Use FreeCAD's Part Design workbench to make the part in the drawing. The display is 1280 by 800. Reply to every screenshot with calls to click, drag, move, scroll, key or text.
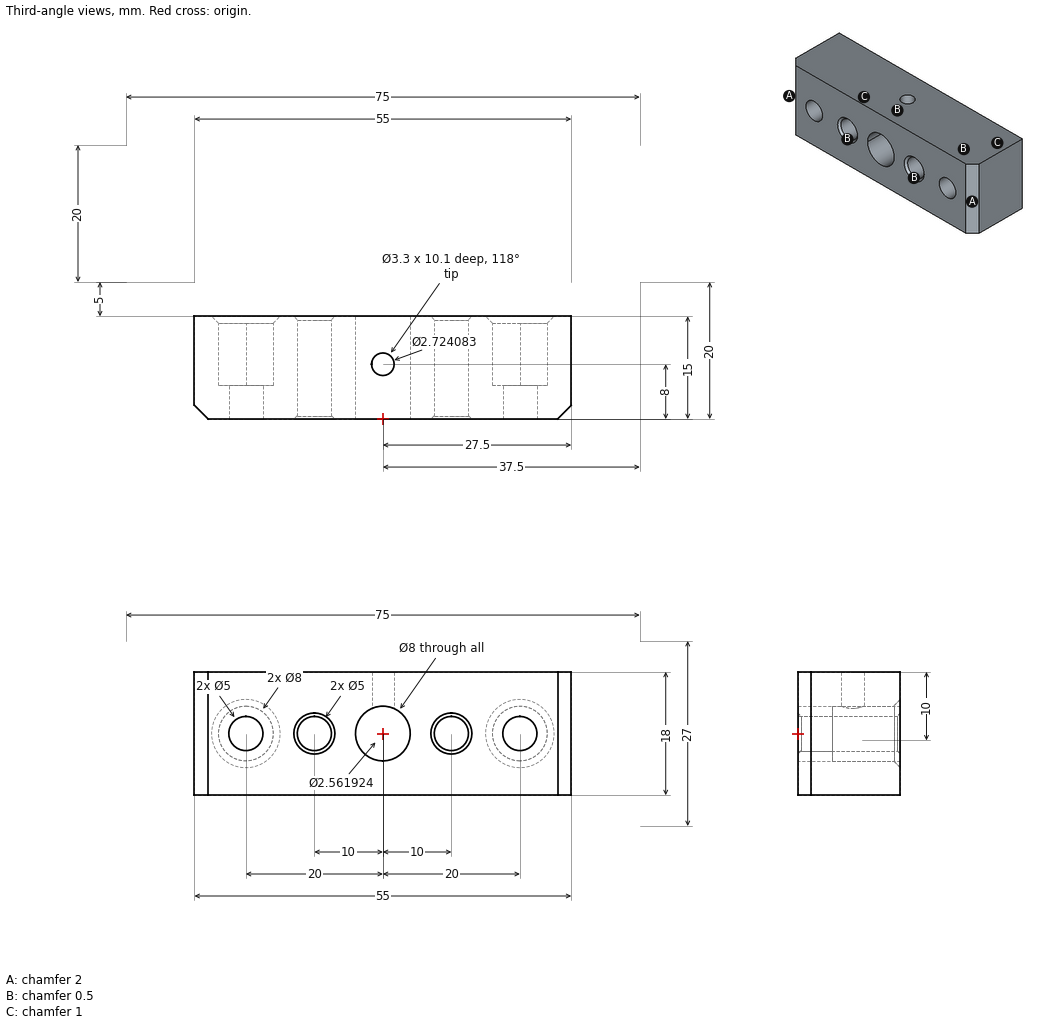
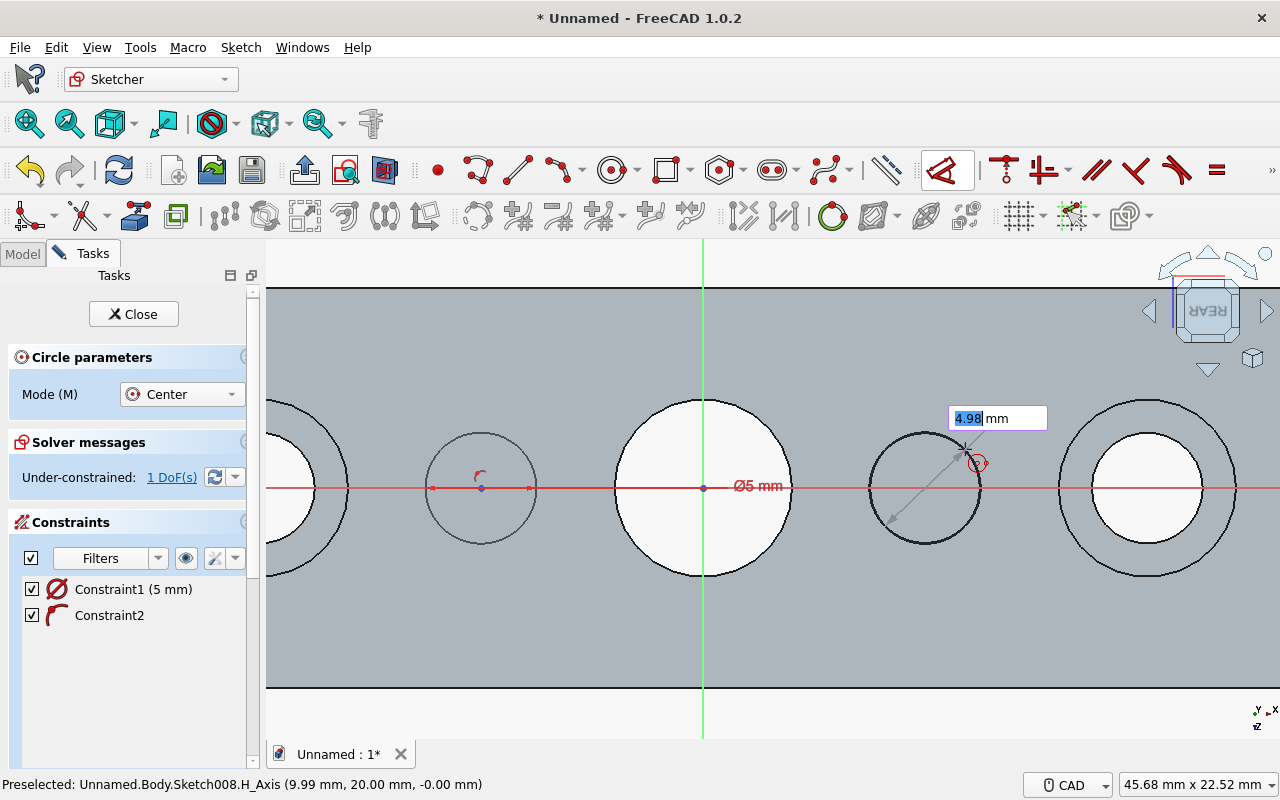
text(5)
key(Return)
key(Escape)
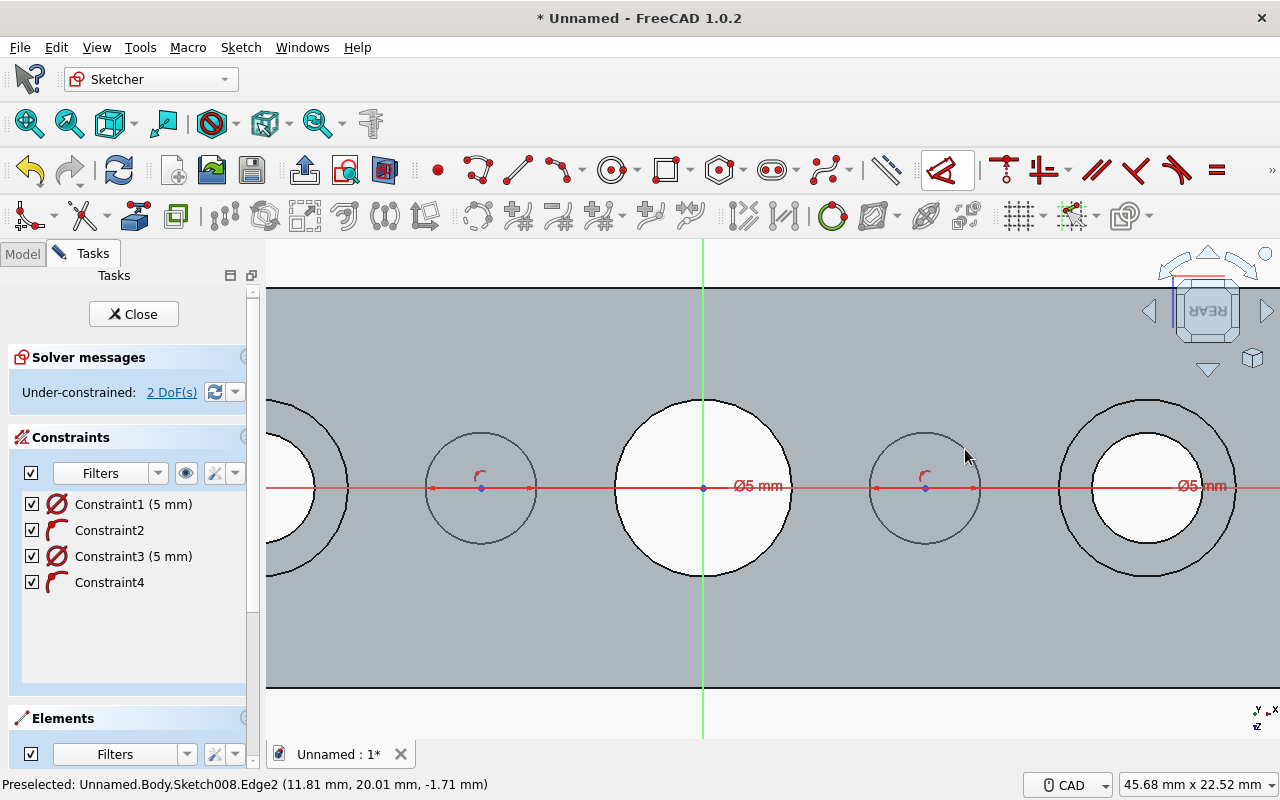
click(481, 488)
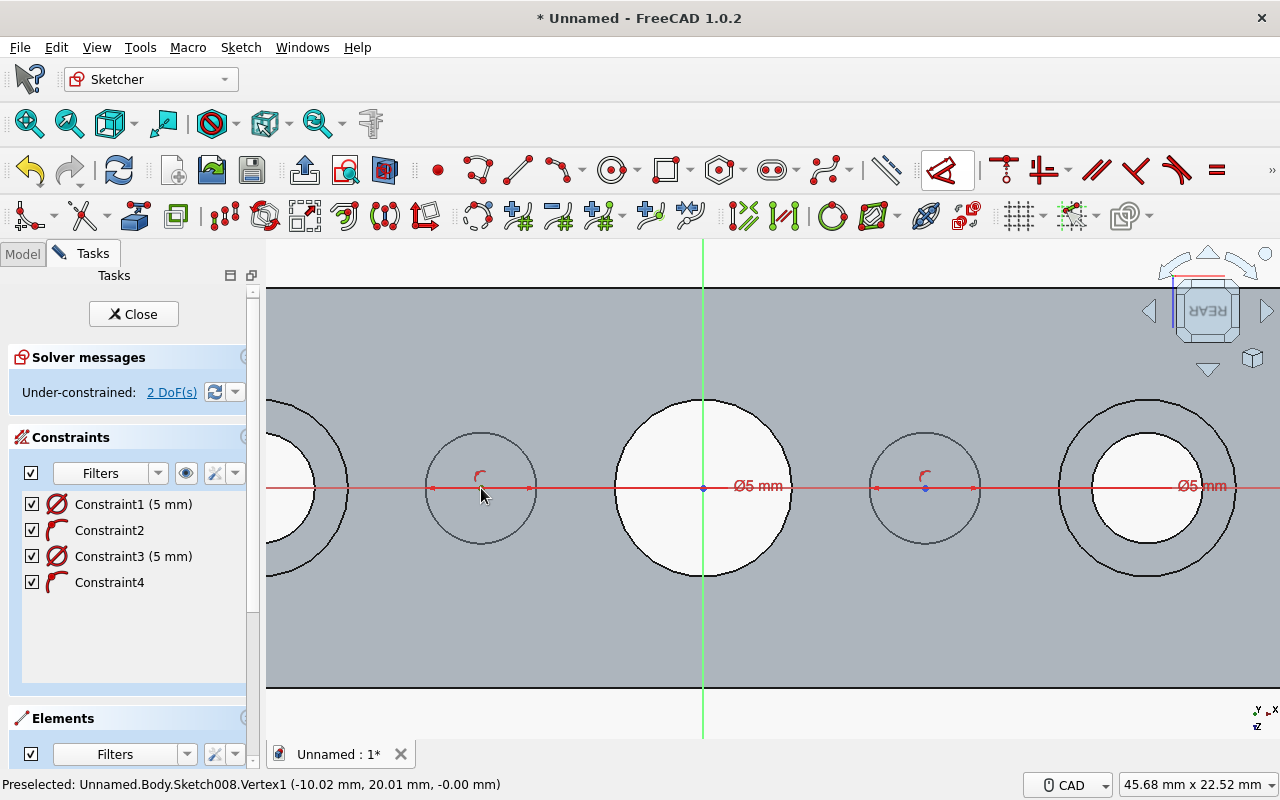
click(968, 170)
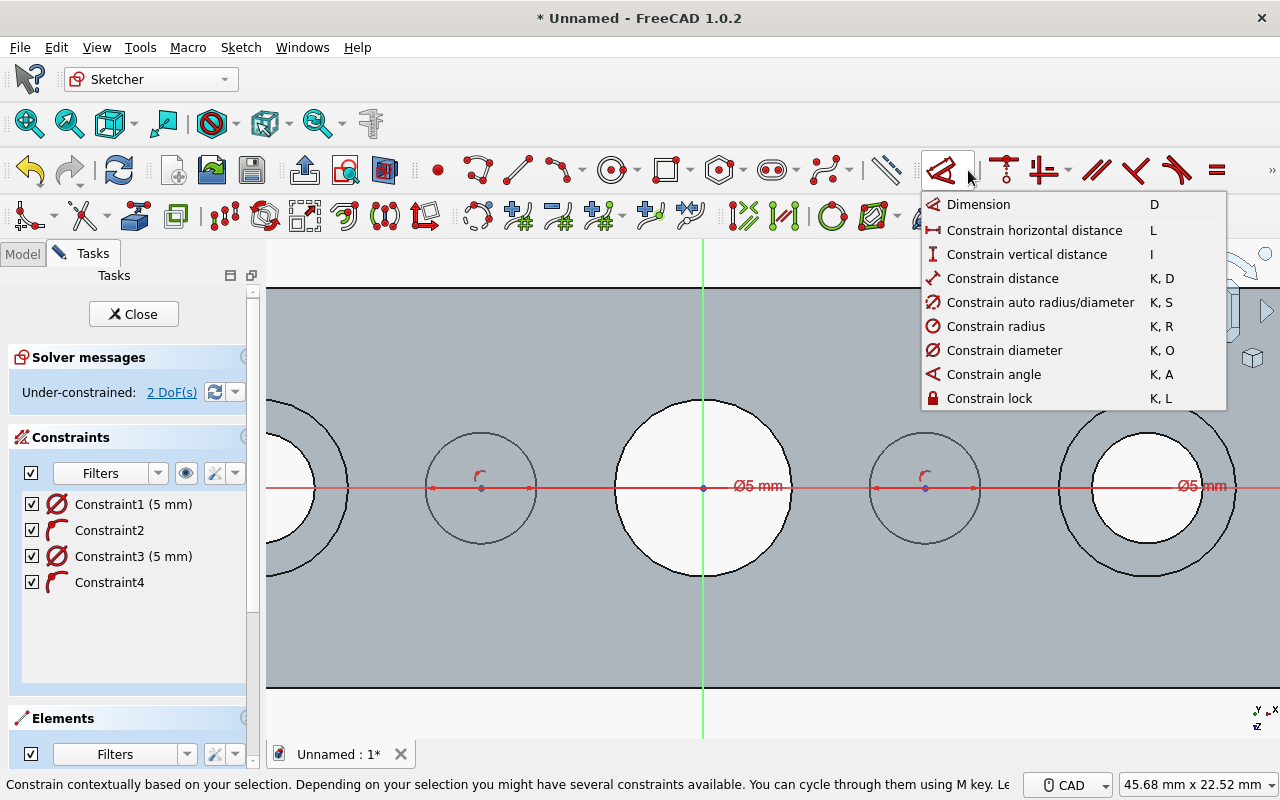
click(1074, 230)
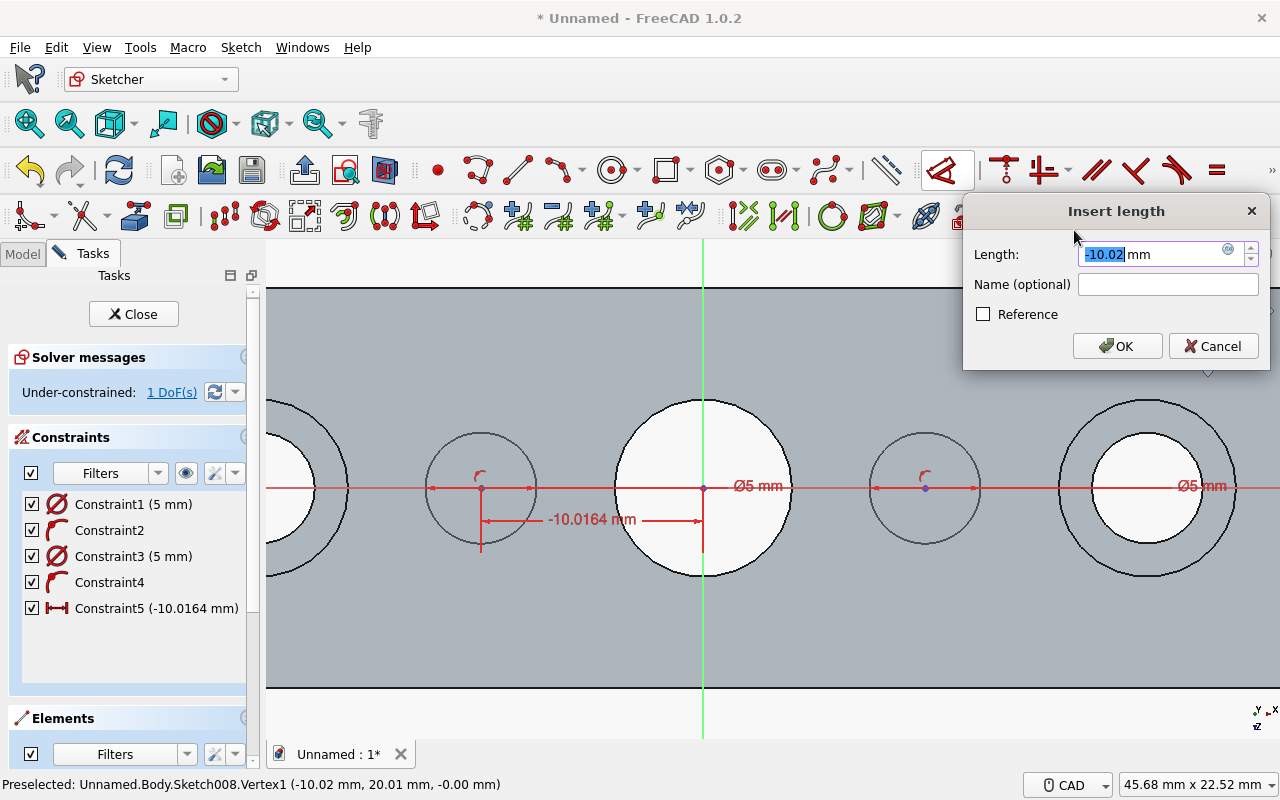
text(-10)
key(Return)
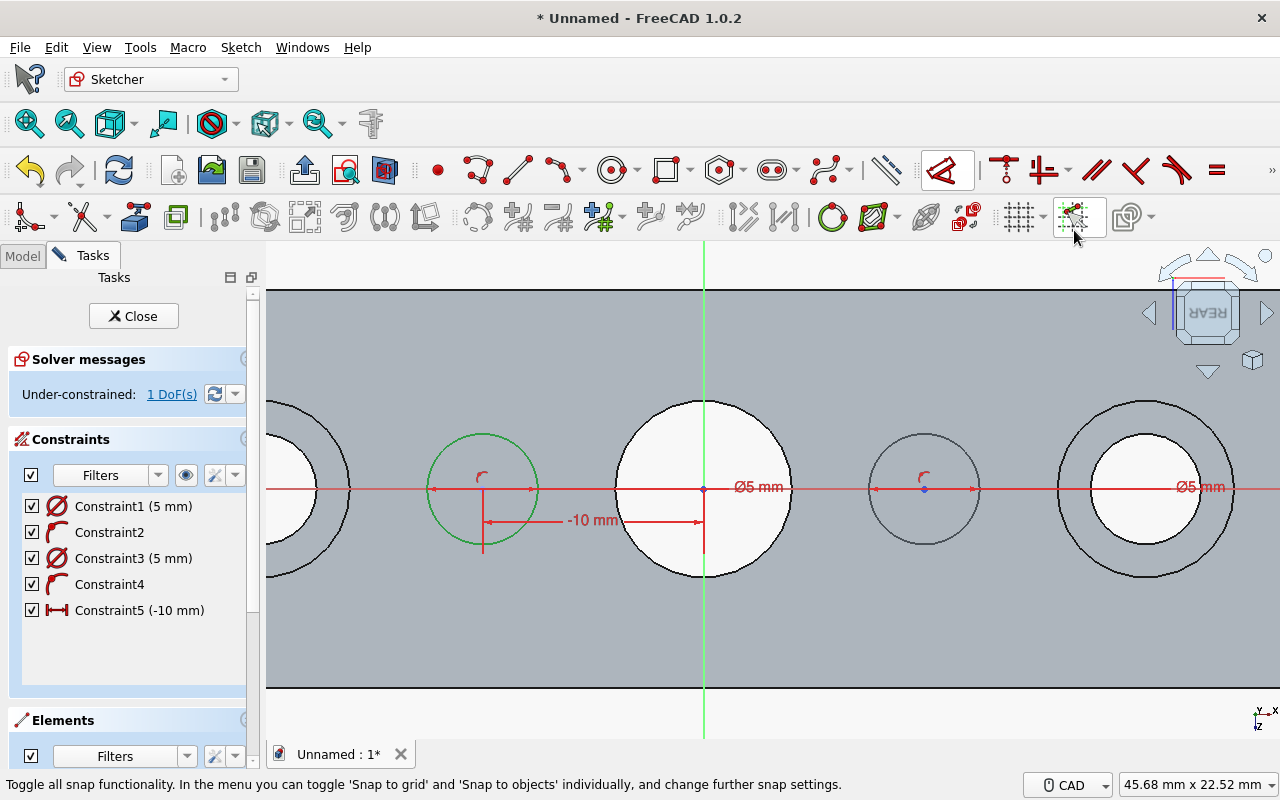
click(924, 489)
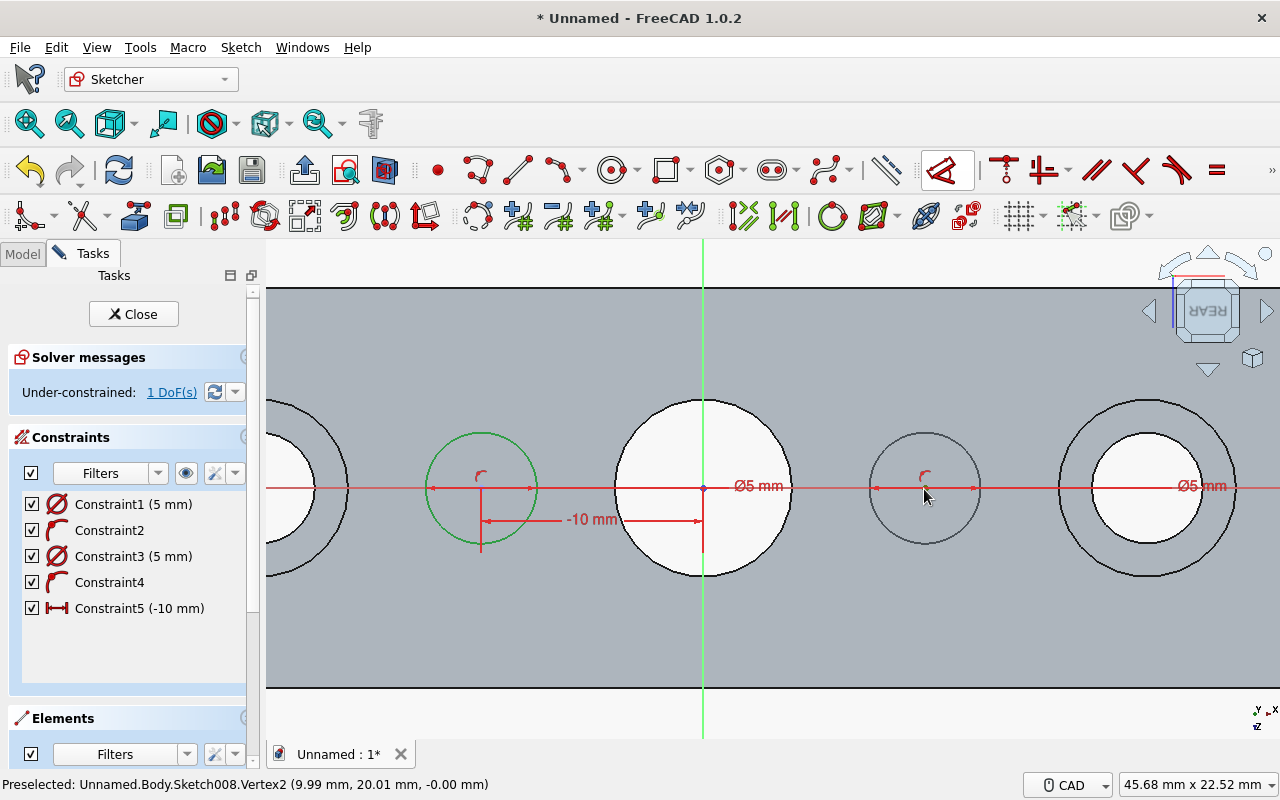
click(968, 170)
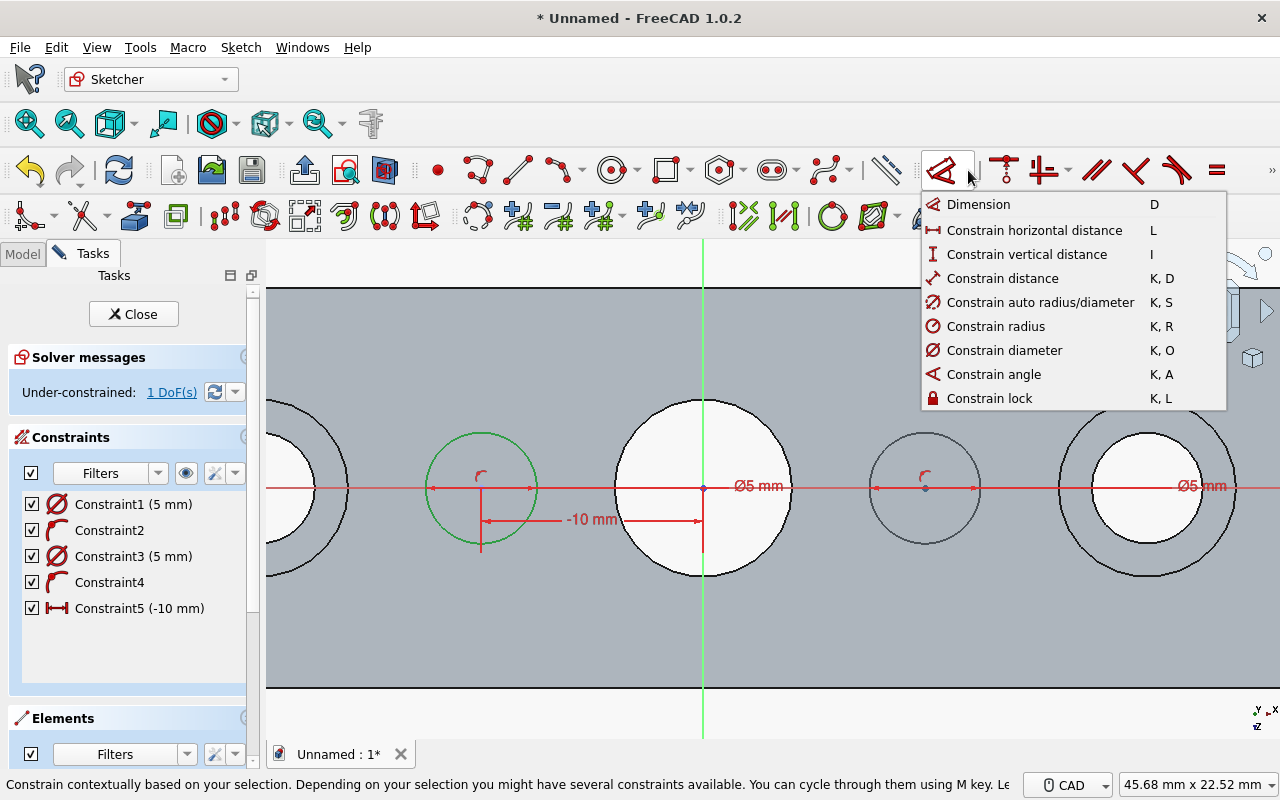
click(1074, 230)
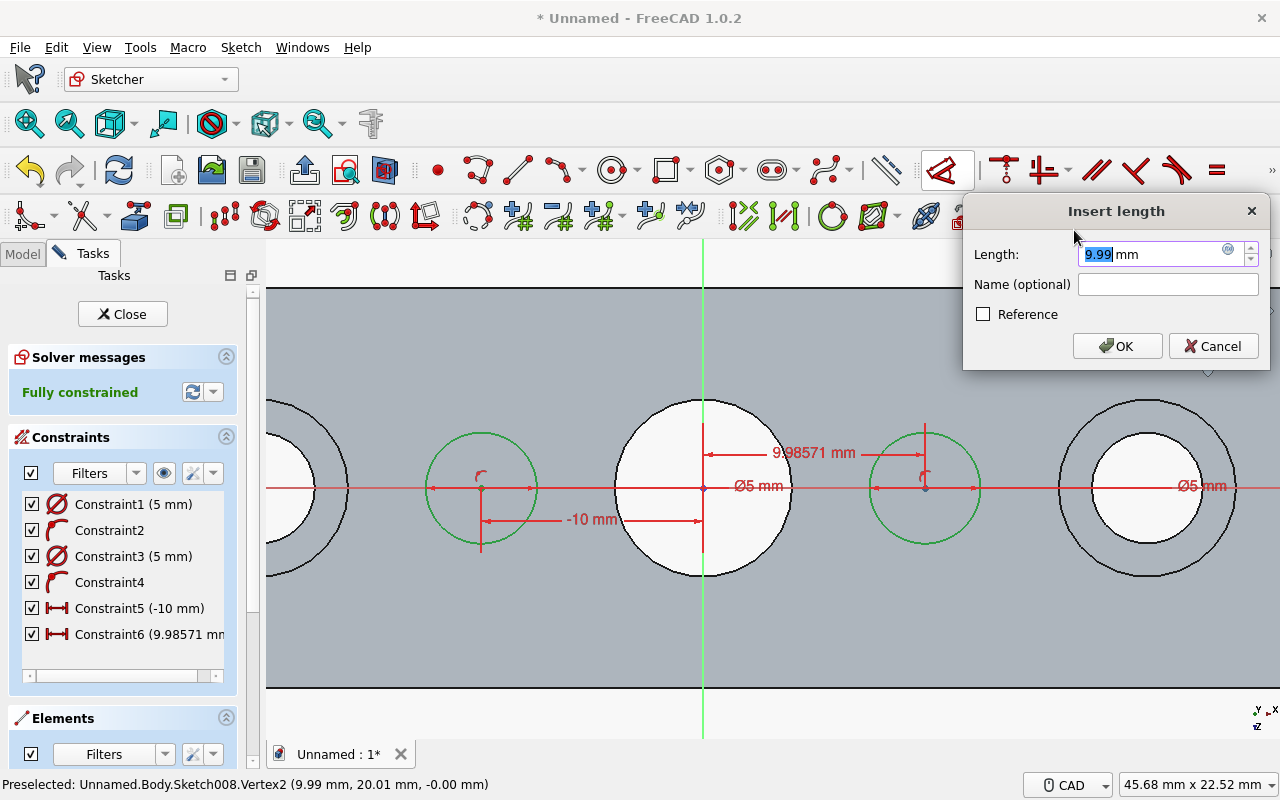
text(10)
key(Return)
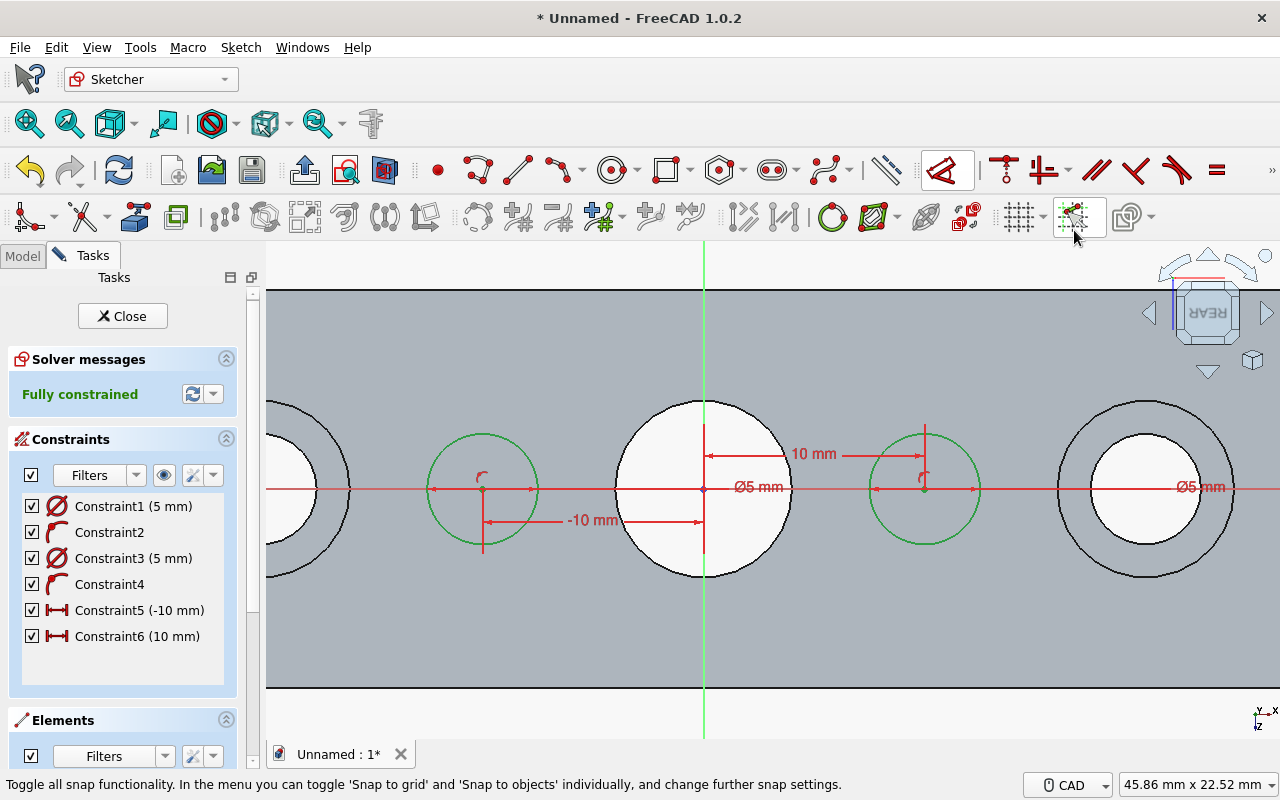
click(123, 316)